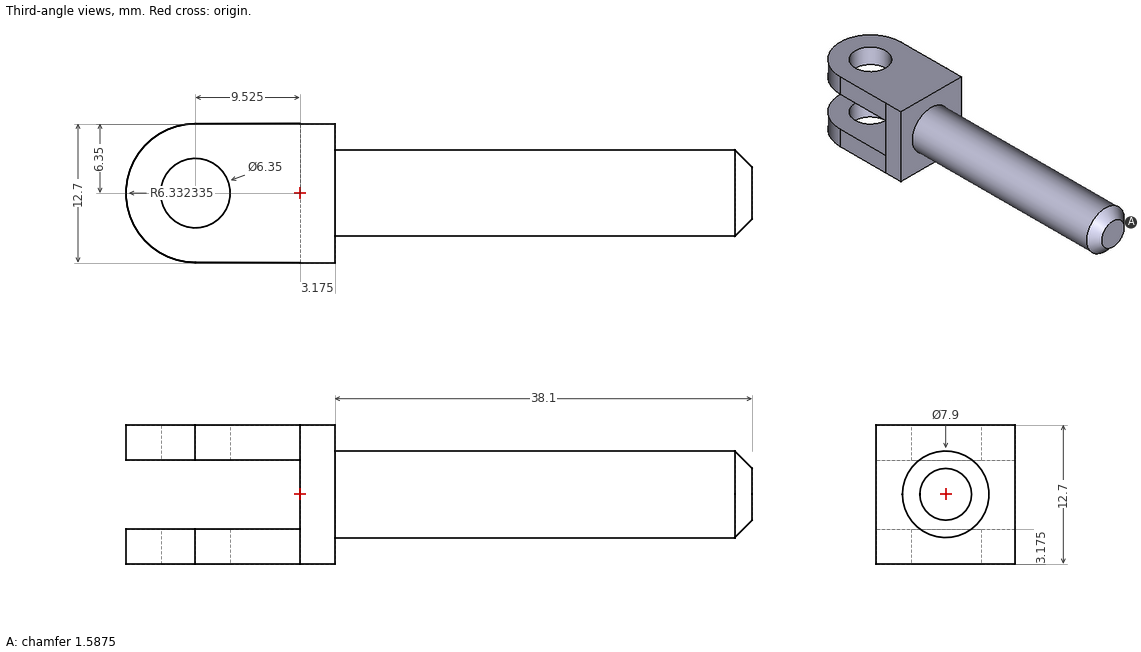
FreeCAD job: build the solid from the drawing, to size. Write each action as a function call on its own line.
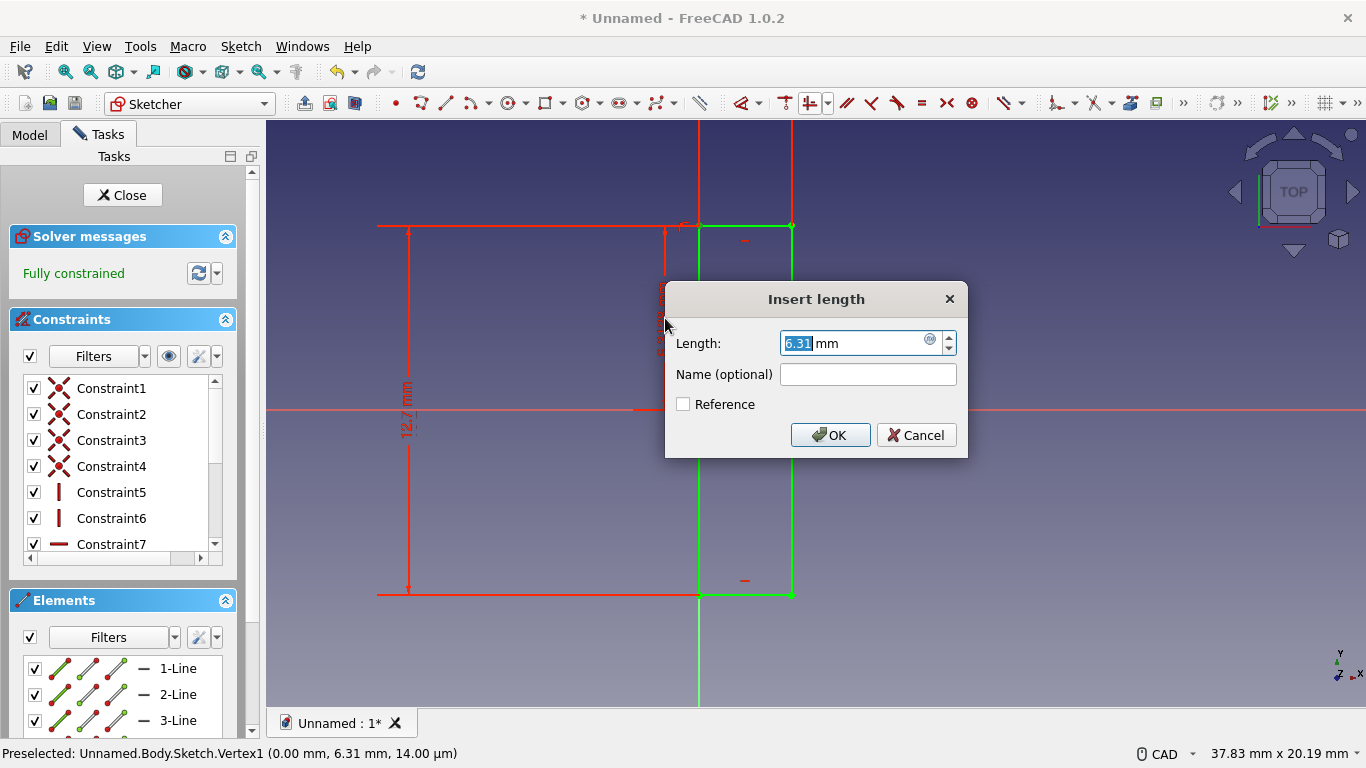
text(6.35)
key(Return)
key(Escape)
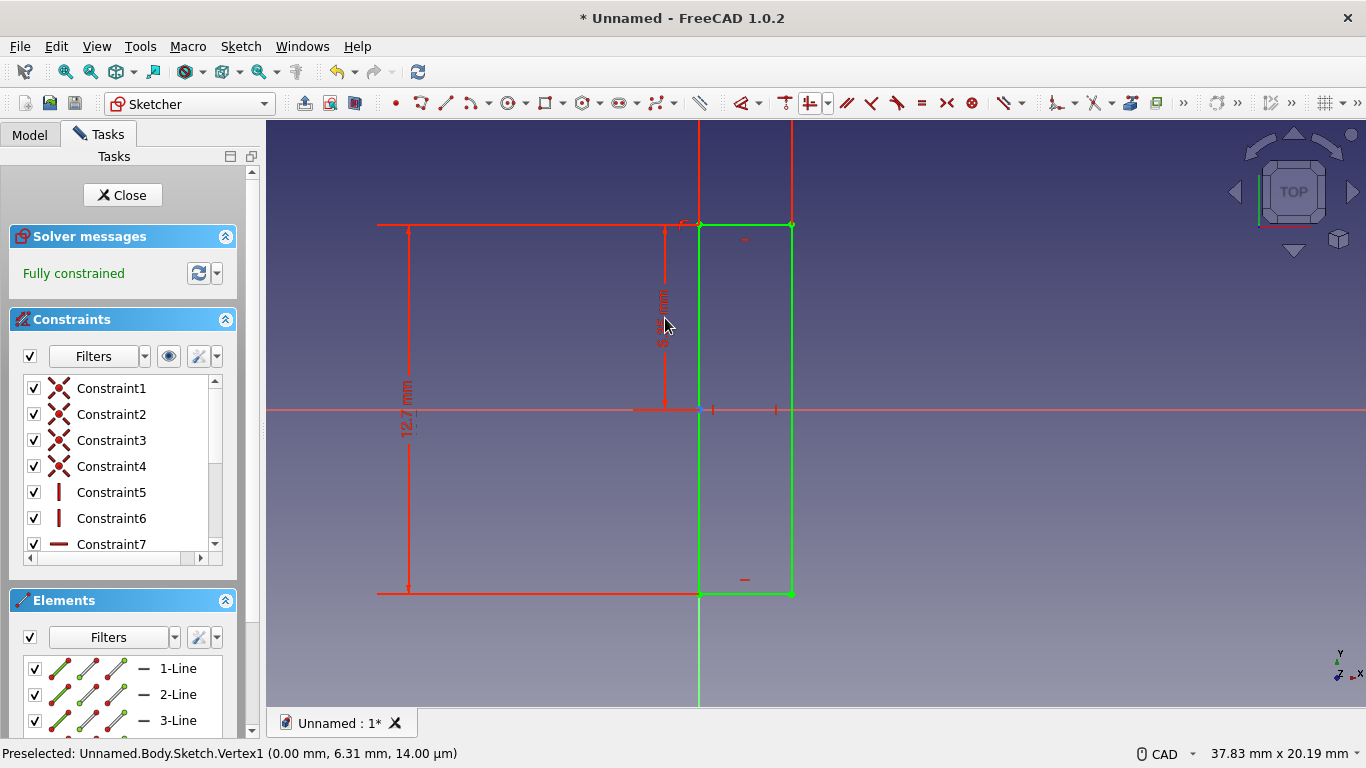
click(123, 195)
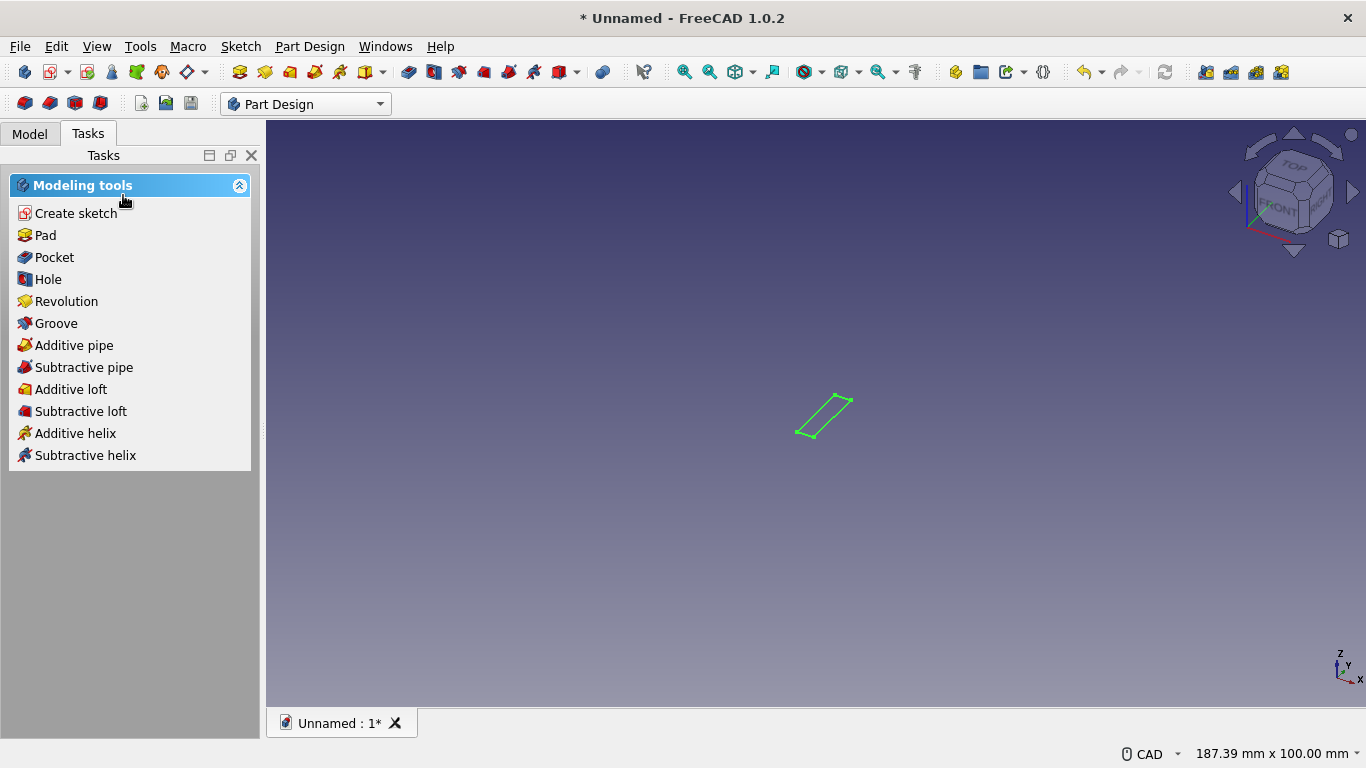
click(240, 72)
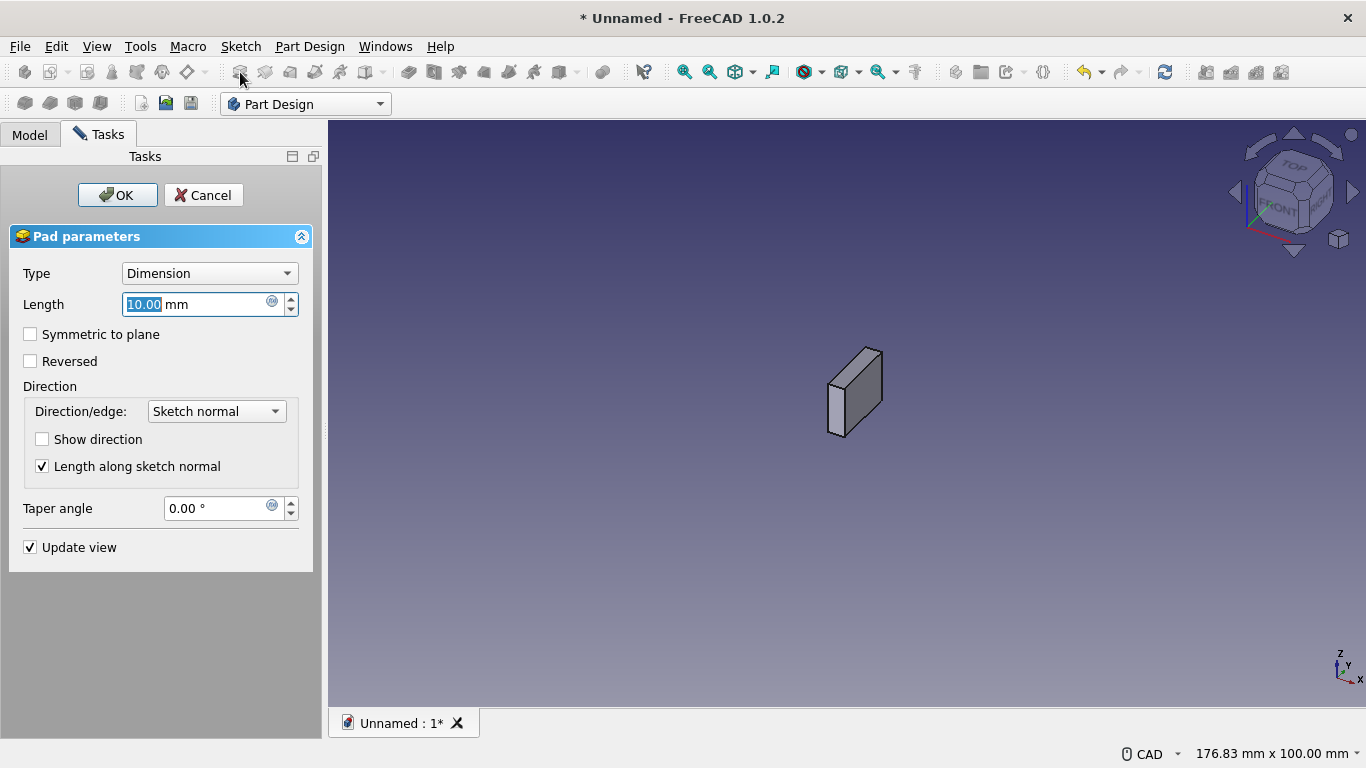
text(12.7)
key(Tab)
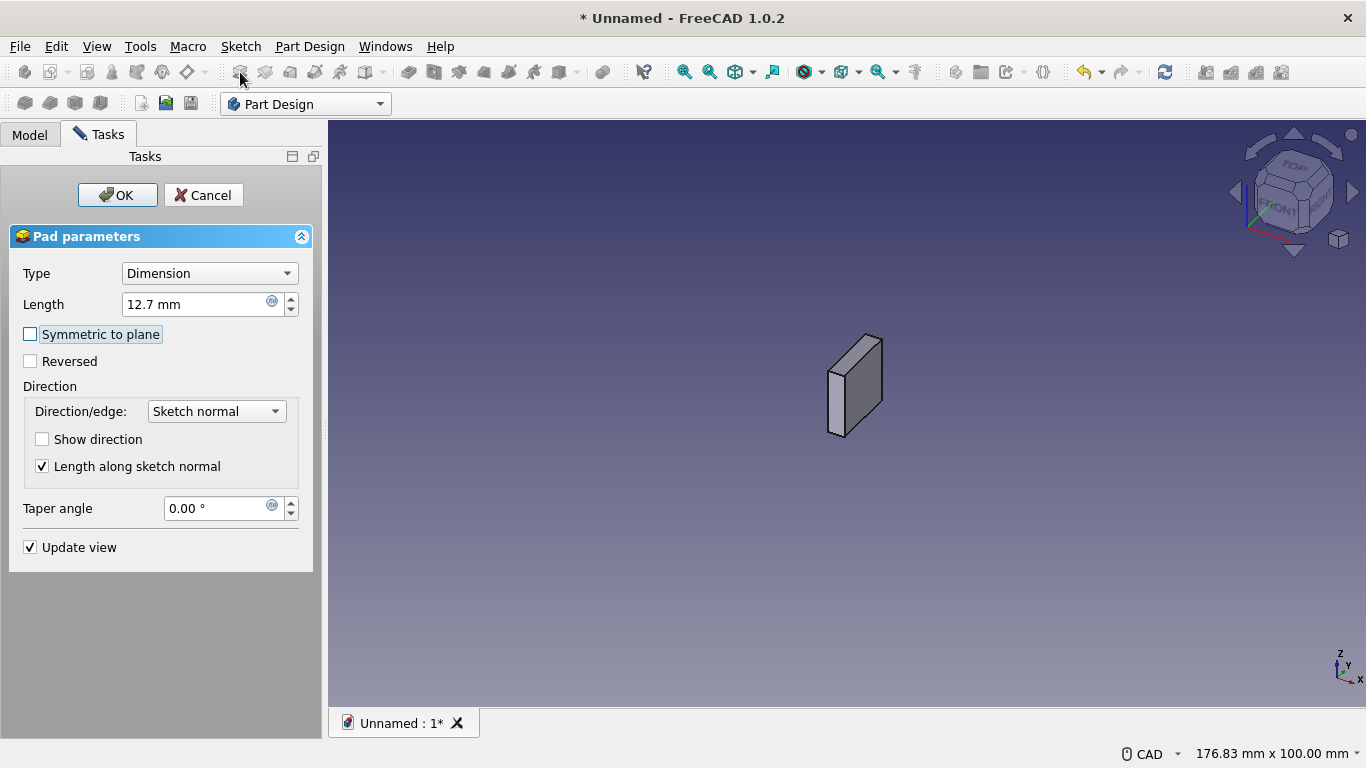
click(31, 334)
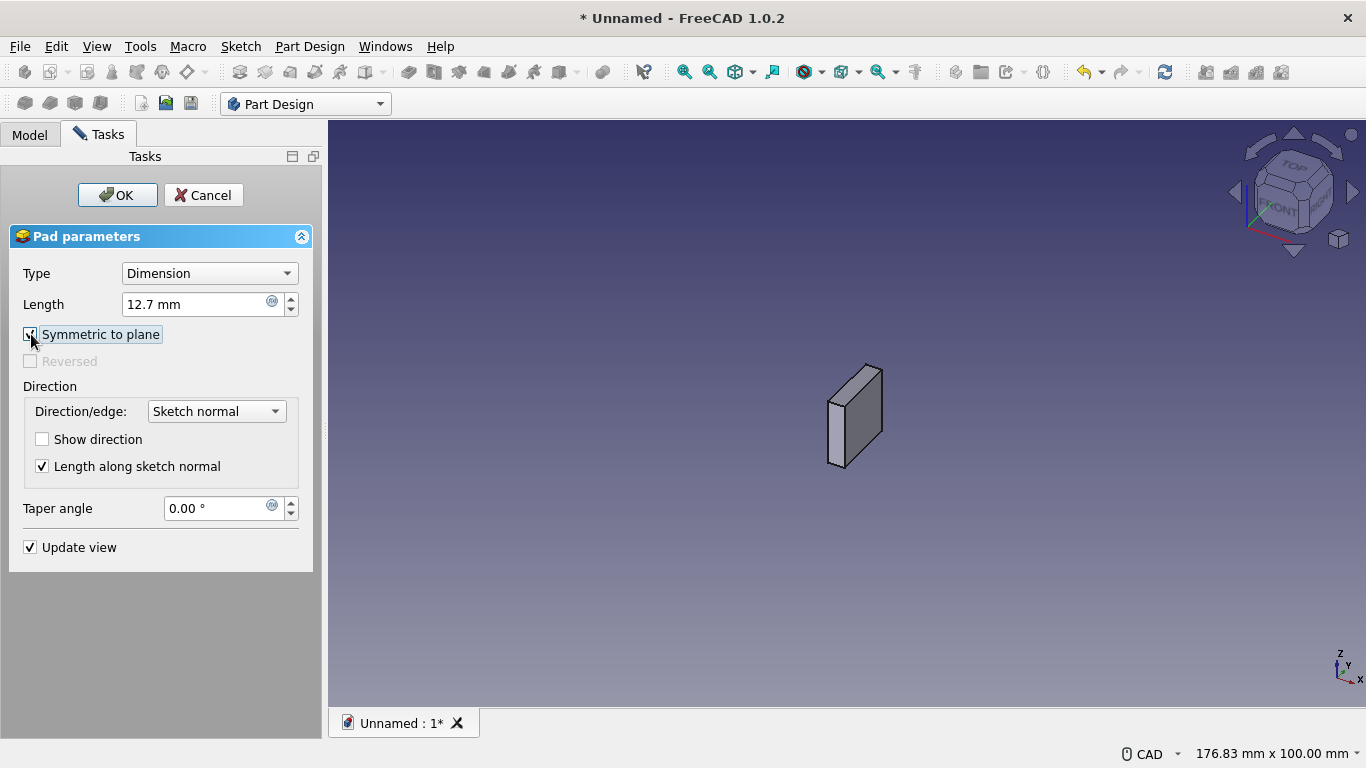
click(118, 195)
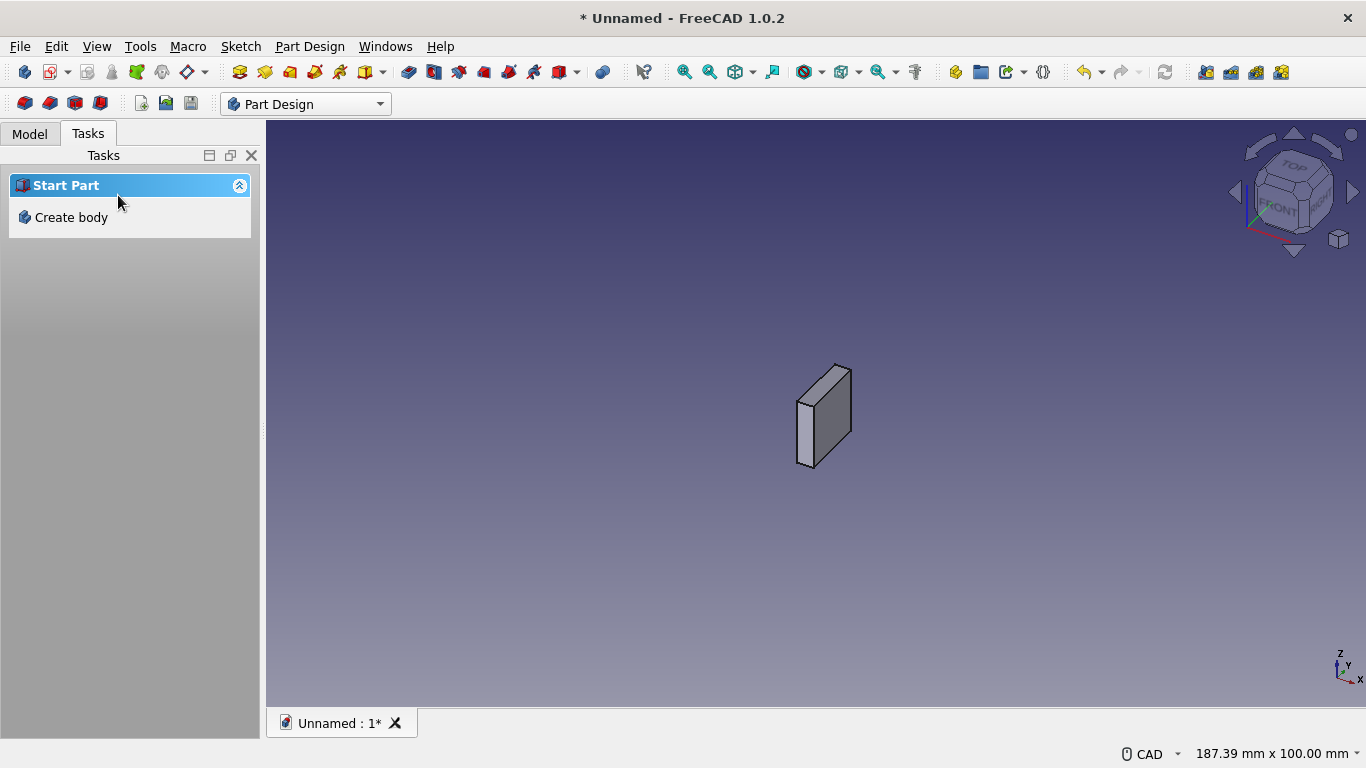
click(685, 72)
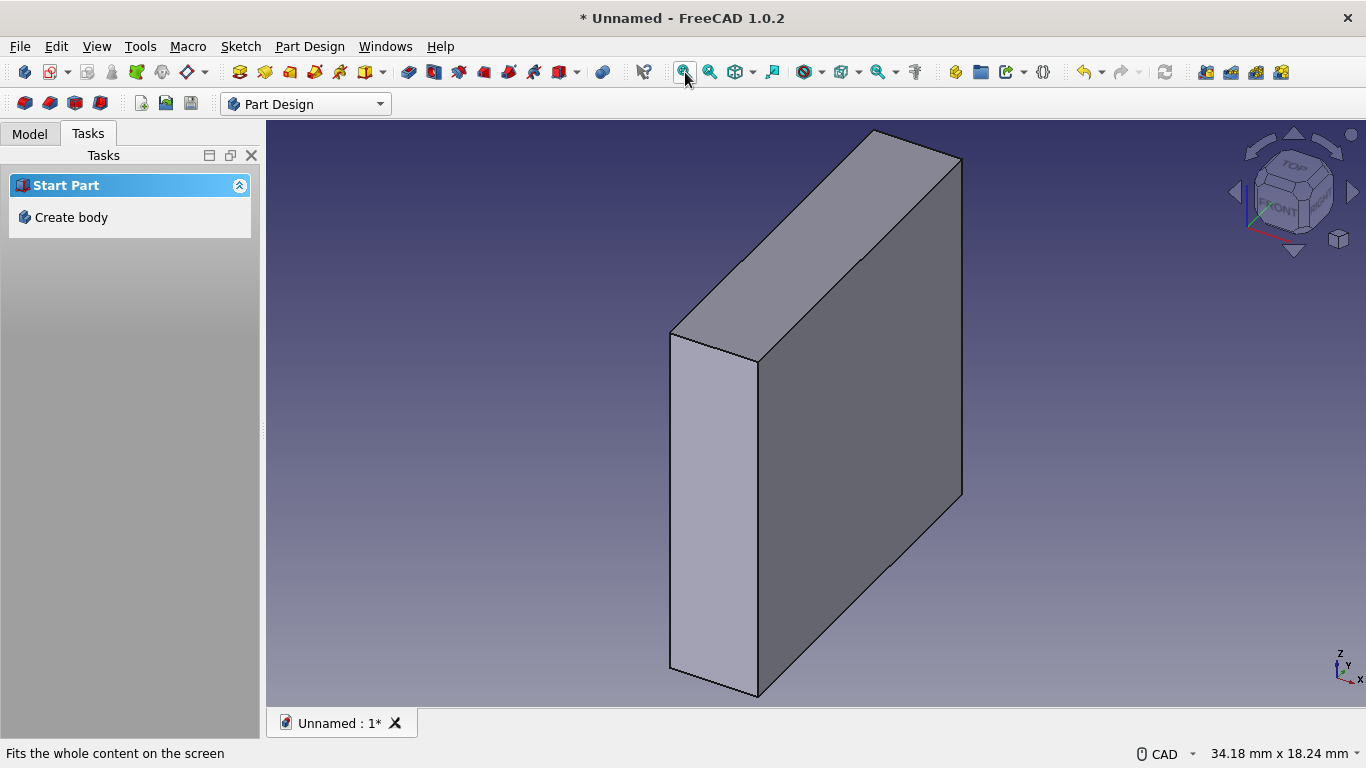
click(860, 427)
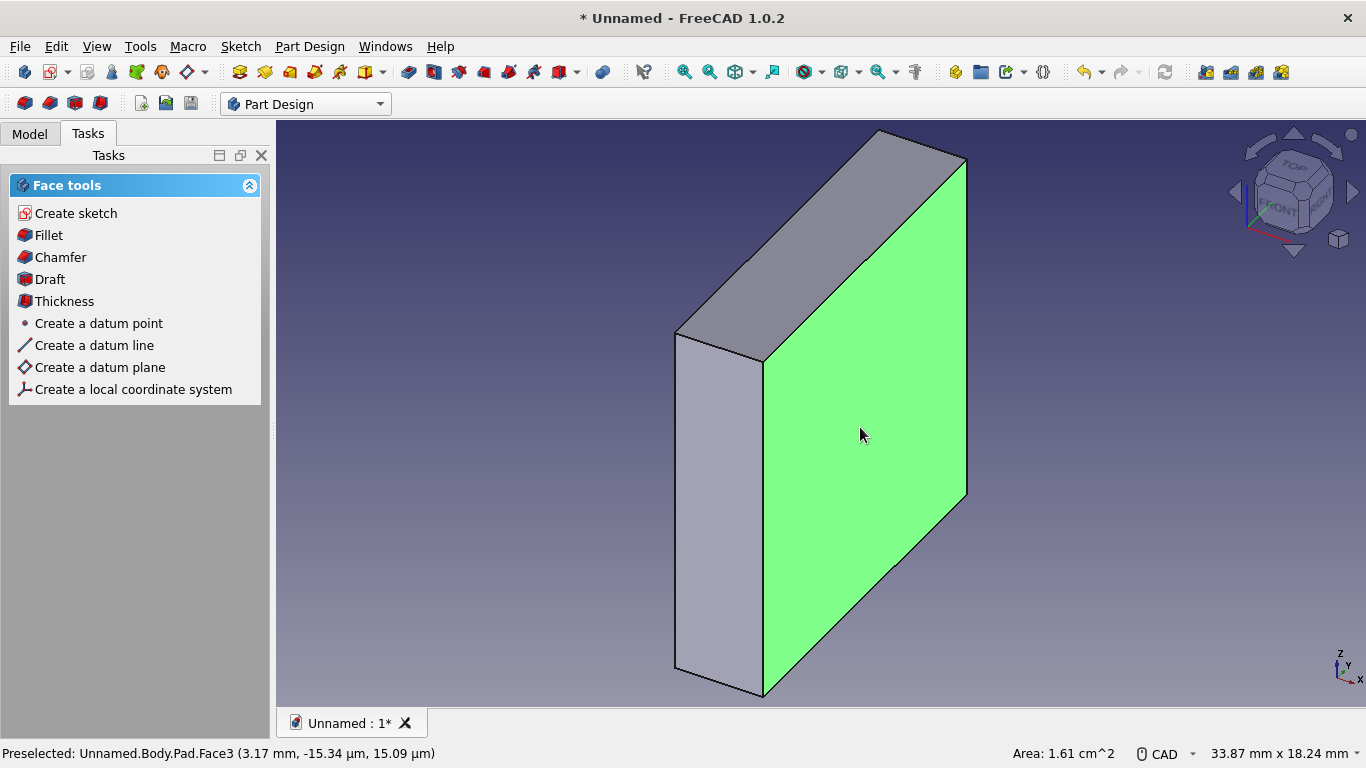
click(50, 72)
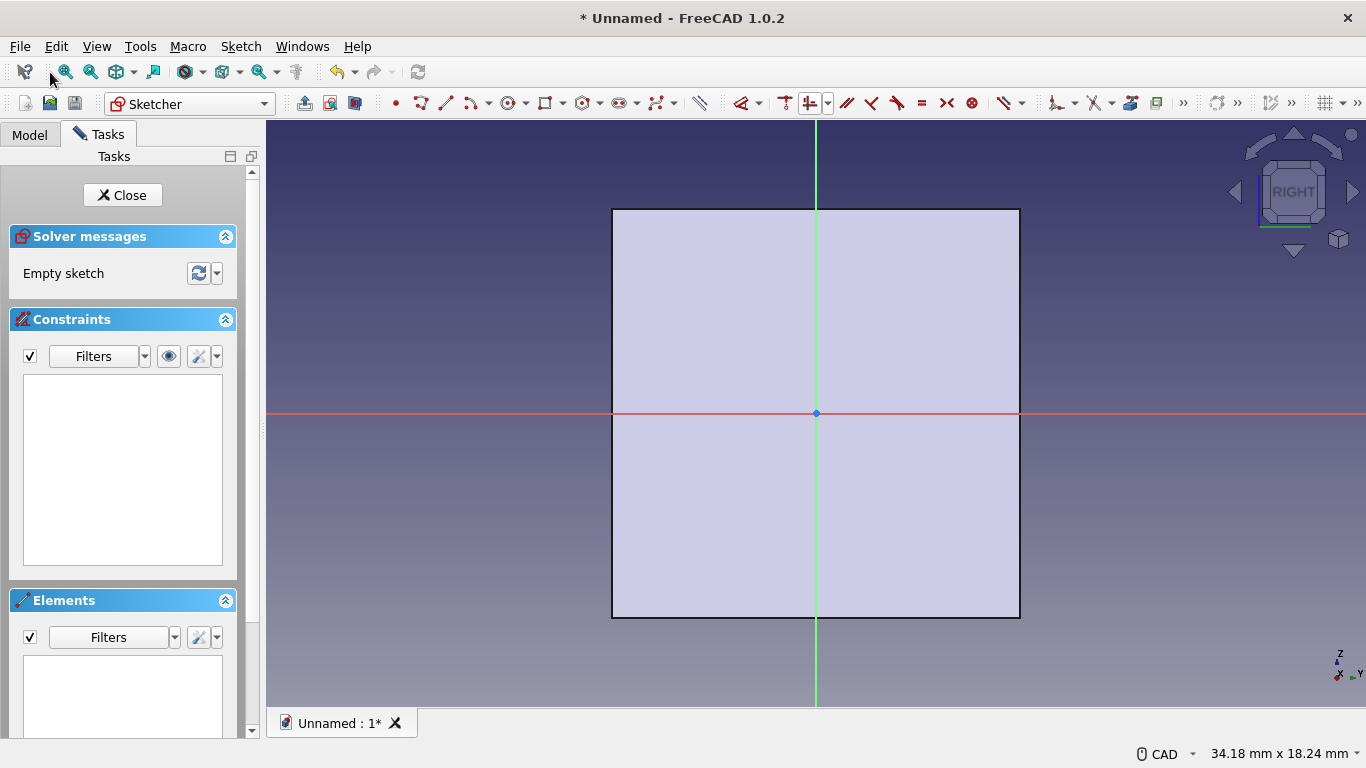
scroll(955, 413, up, 2)